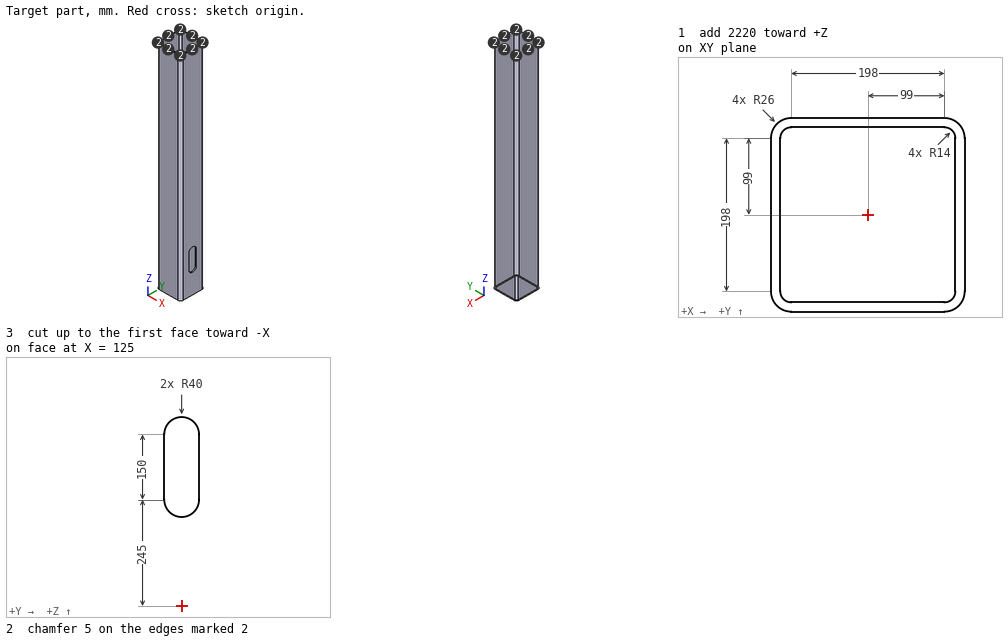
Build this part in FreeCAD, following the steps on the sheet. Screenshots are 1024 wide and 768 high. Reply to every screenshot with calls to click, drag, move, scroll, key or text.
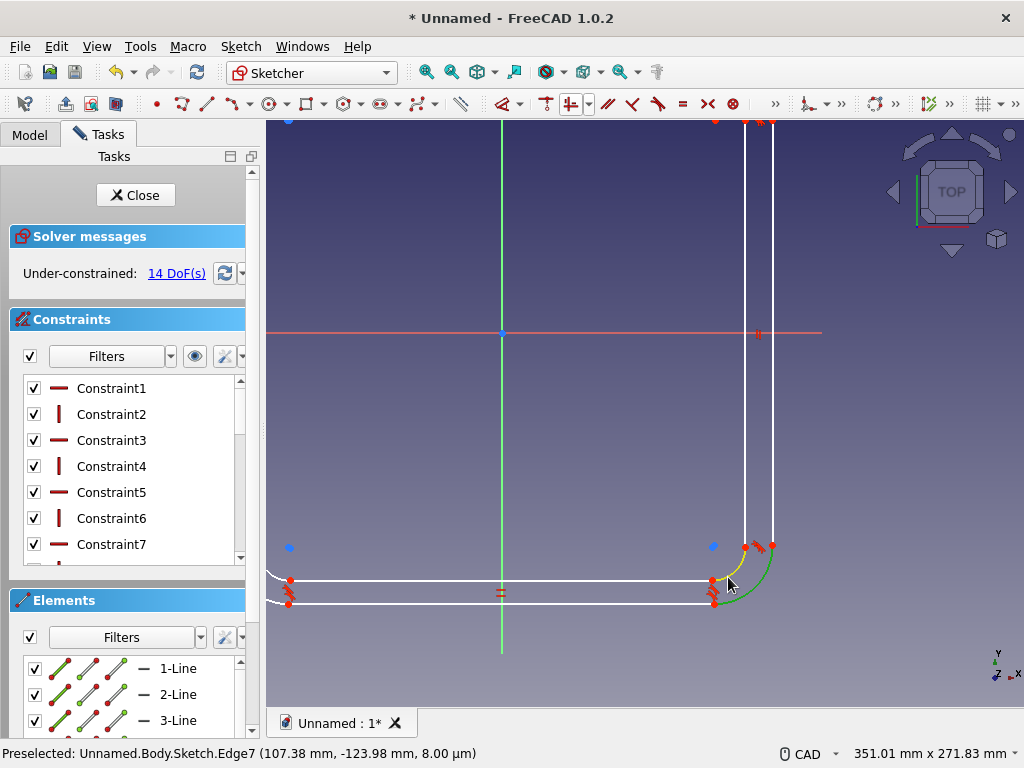
click(727, 577)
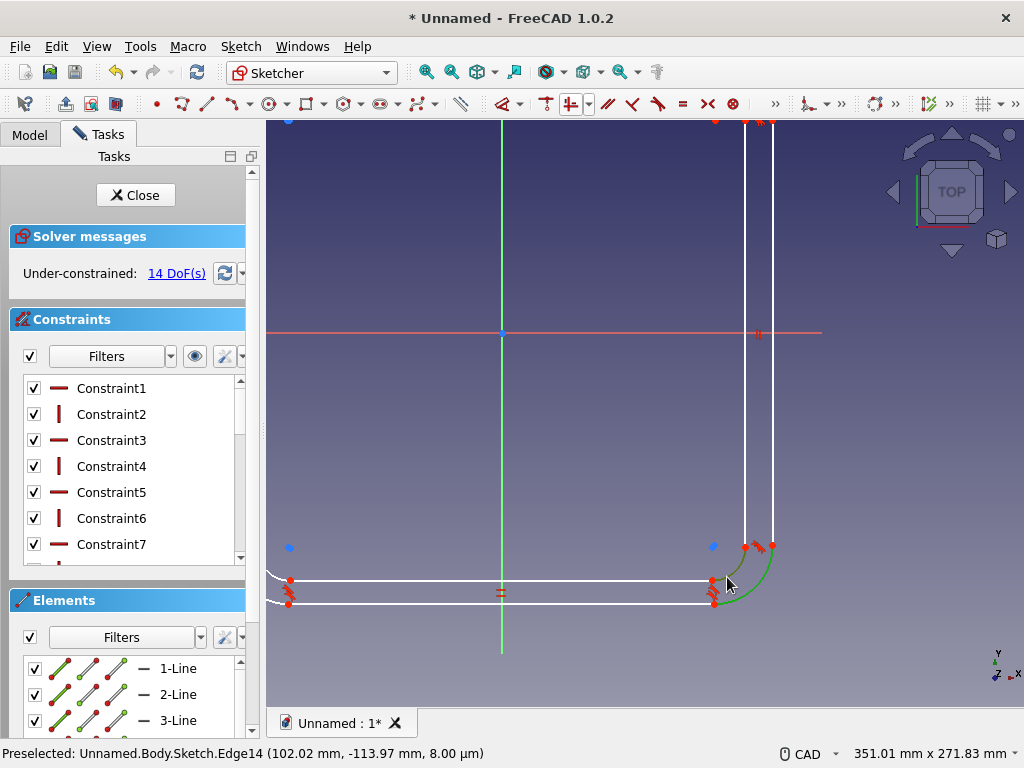
click(546, 104)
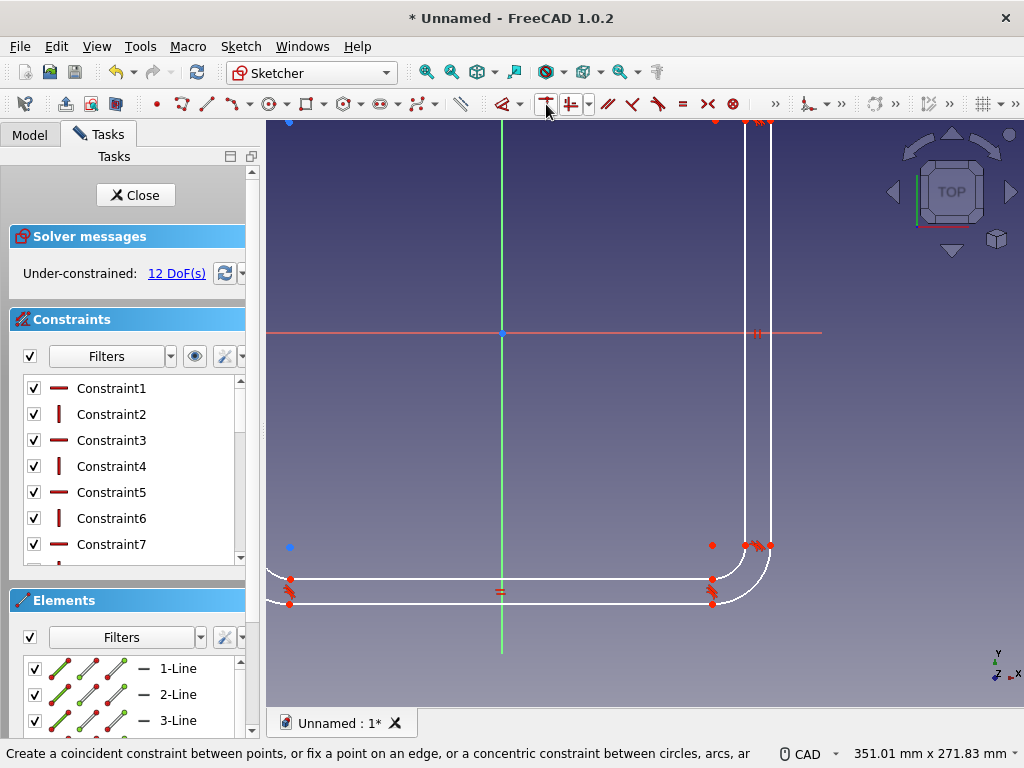
scroll(728, 577, down, 2)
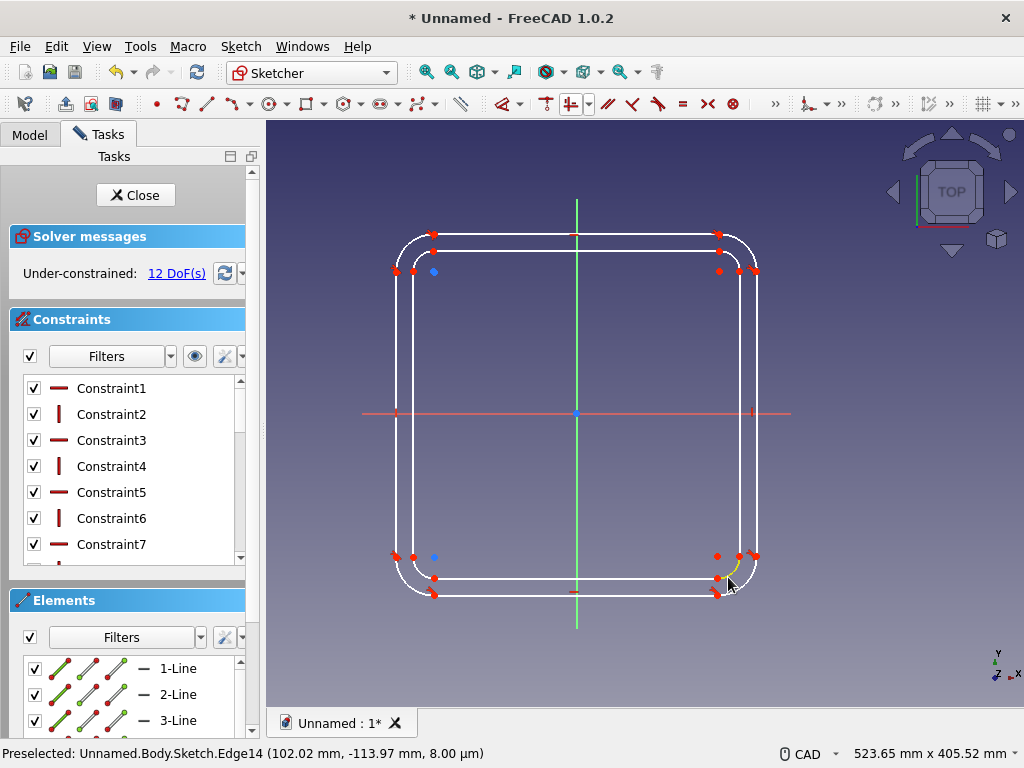
click(400, 575)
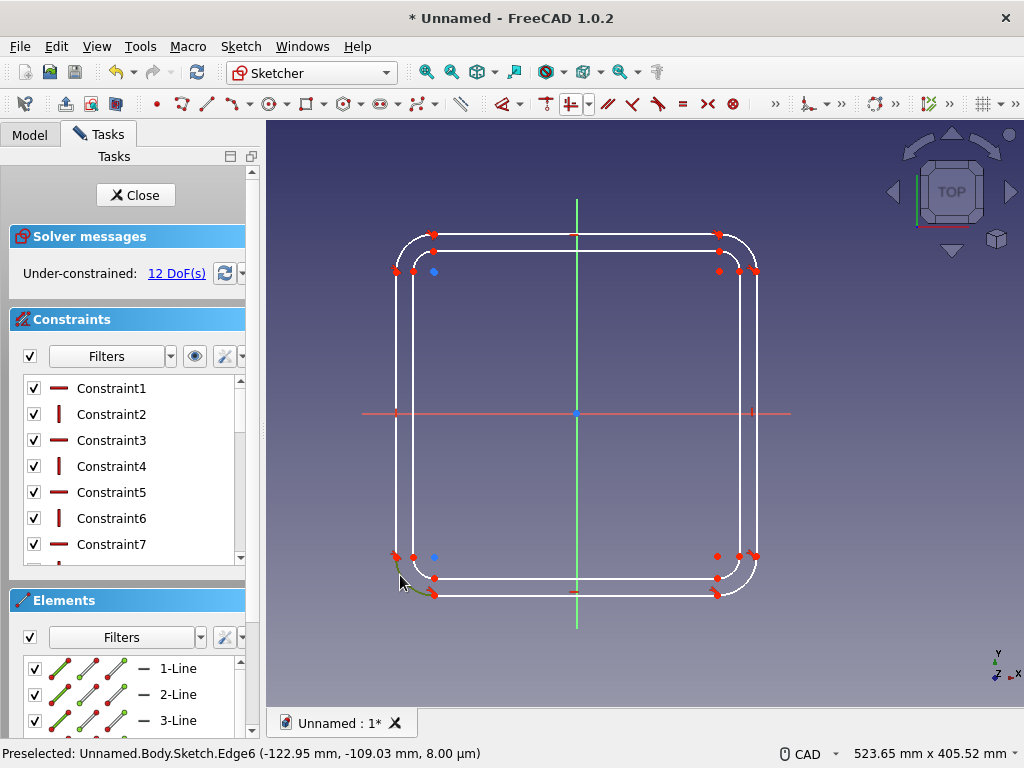
scroll(416, 567, up, 2)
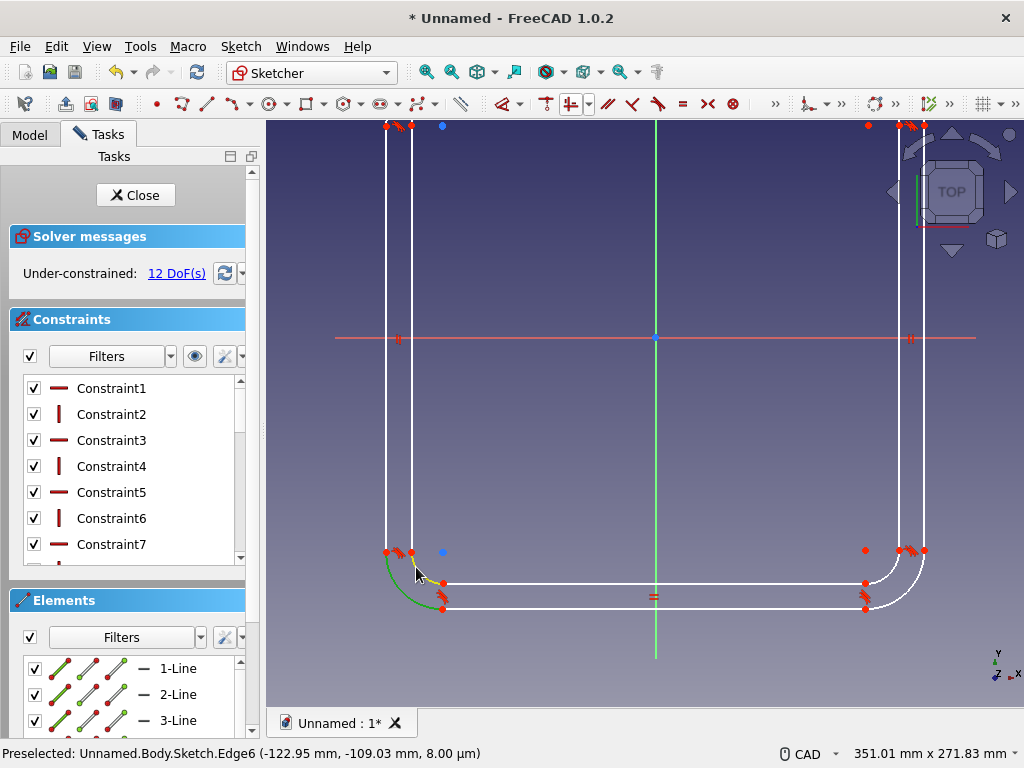
click(415, 567)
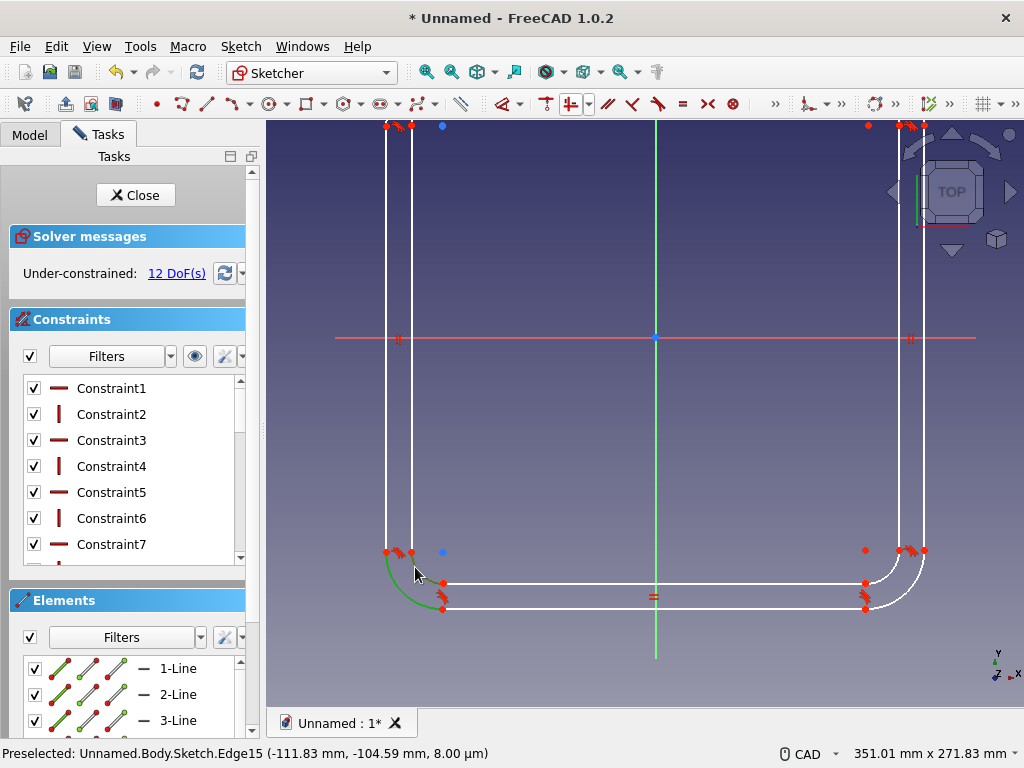
click(546, 104)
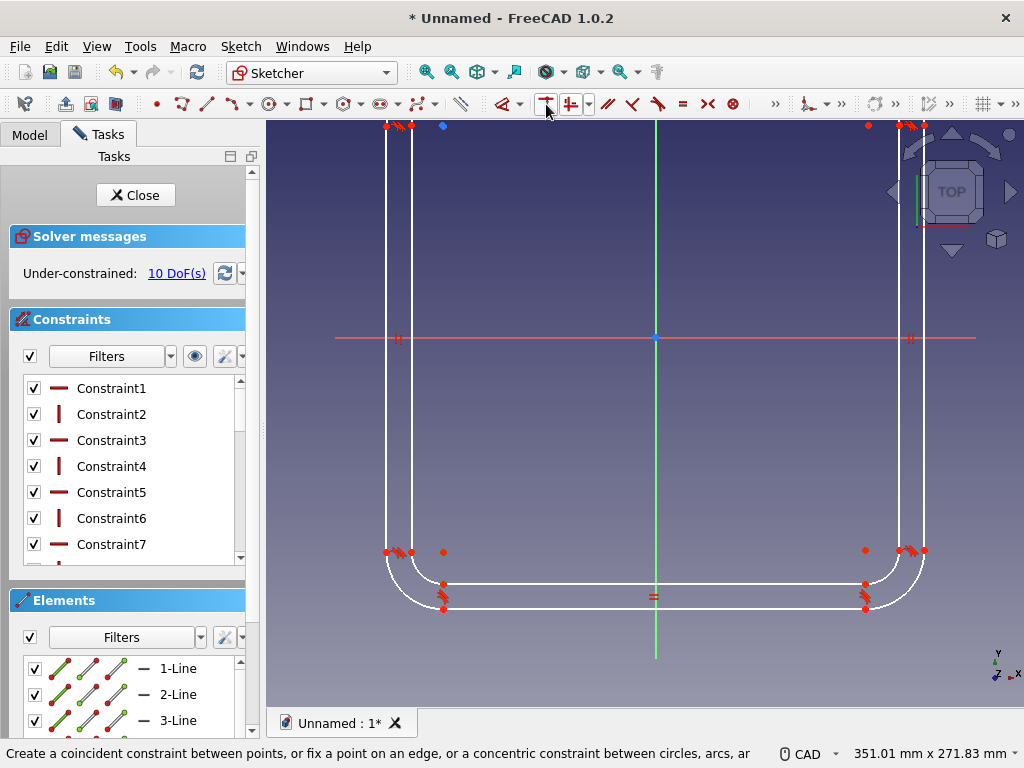
scroll(416, 567, down, 2)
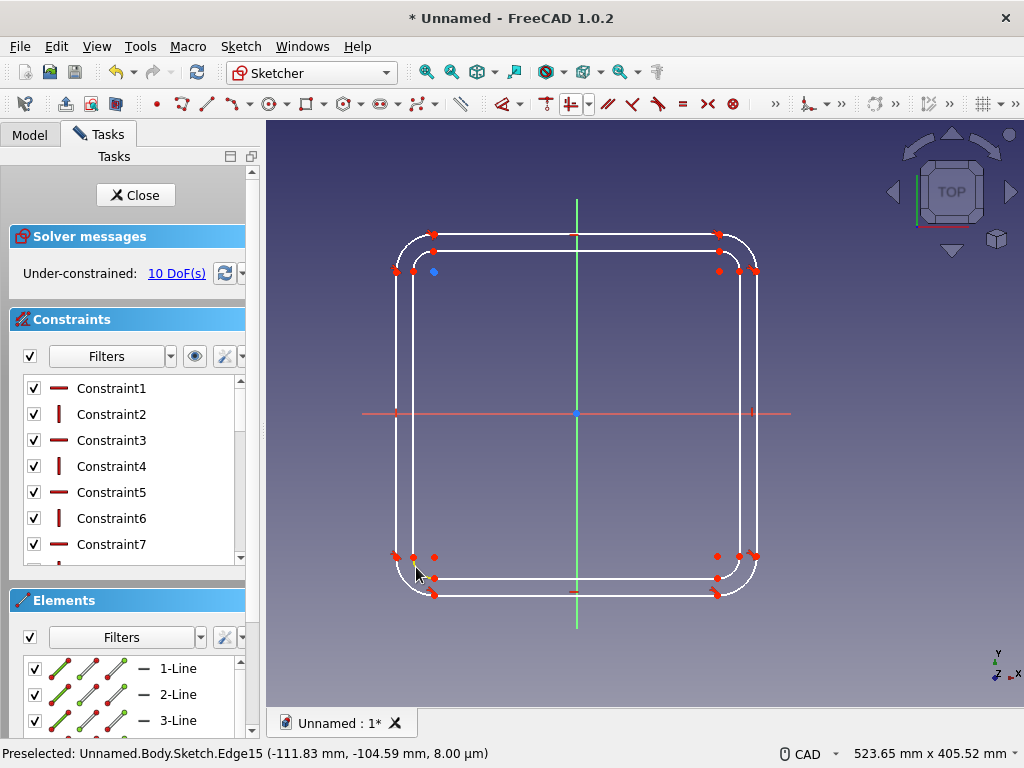
click(417, 238)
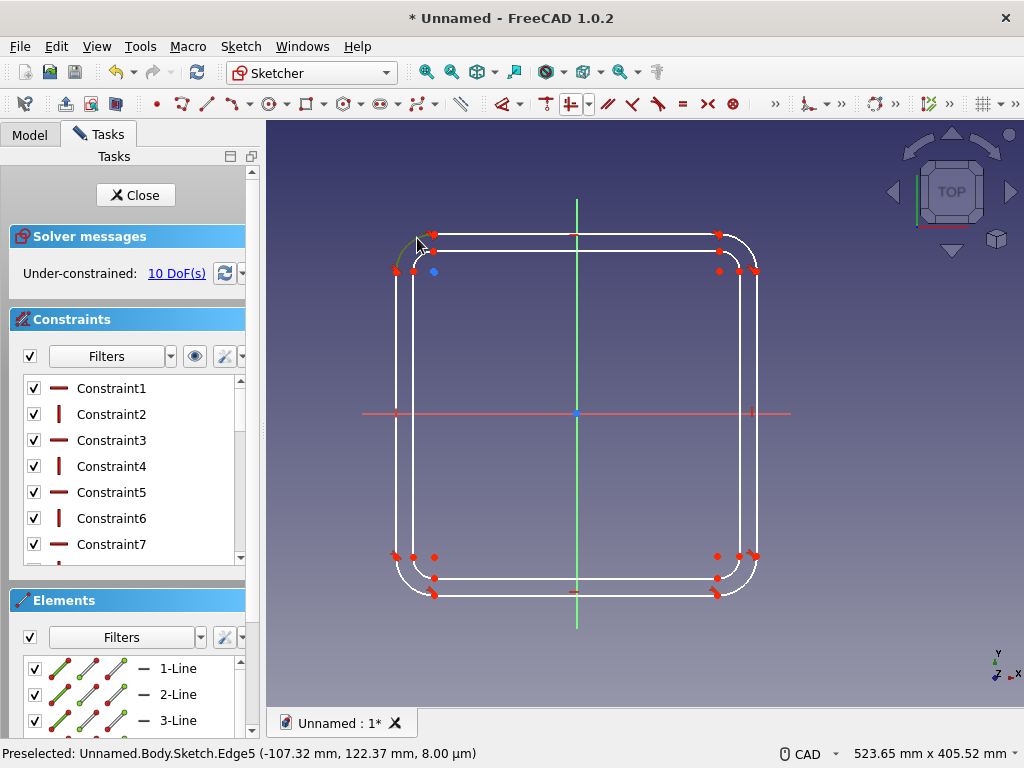
click(400, 575)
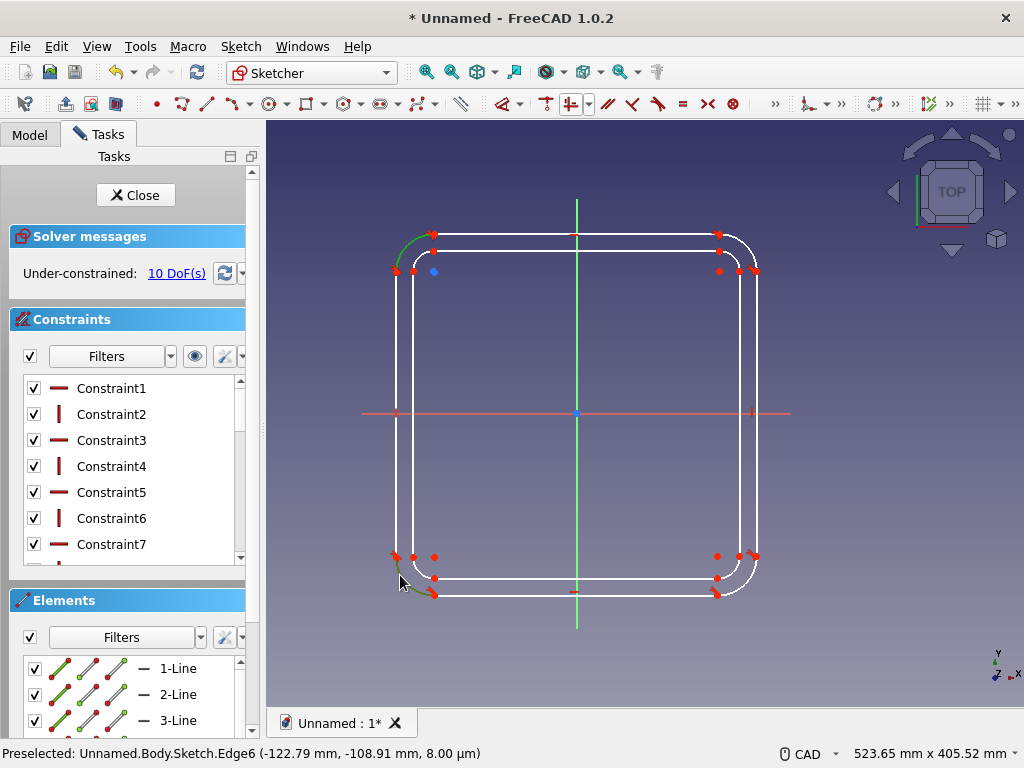
click(735, 591)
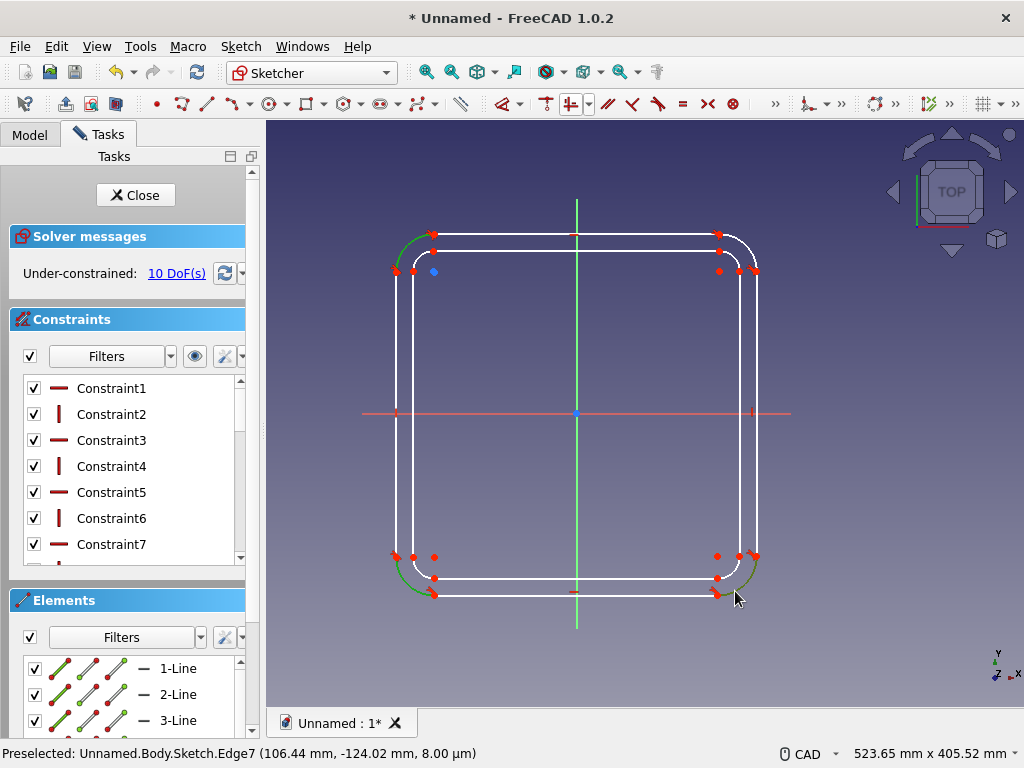
click(753, 255)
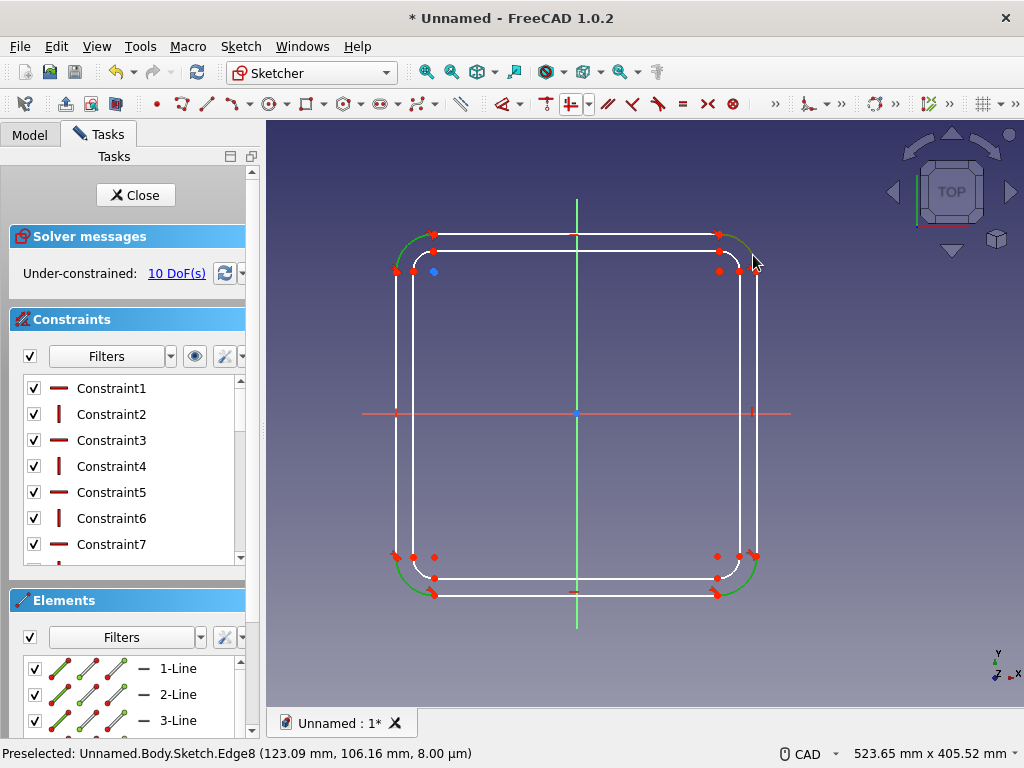
click(683, 104)